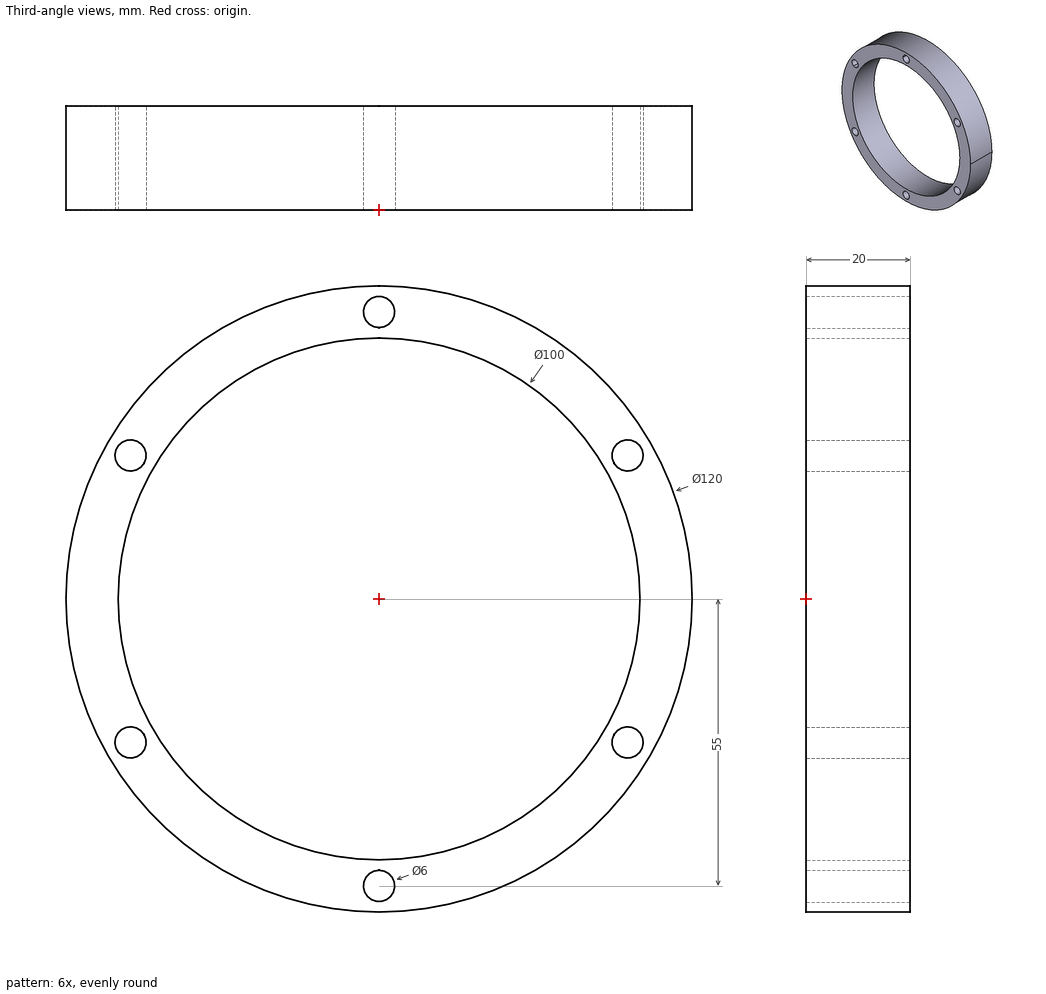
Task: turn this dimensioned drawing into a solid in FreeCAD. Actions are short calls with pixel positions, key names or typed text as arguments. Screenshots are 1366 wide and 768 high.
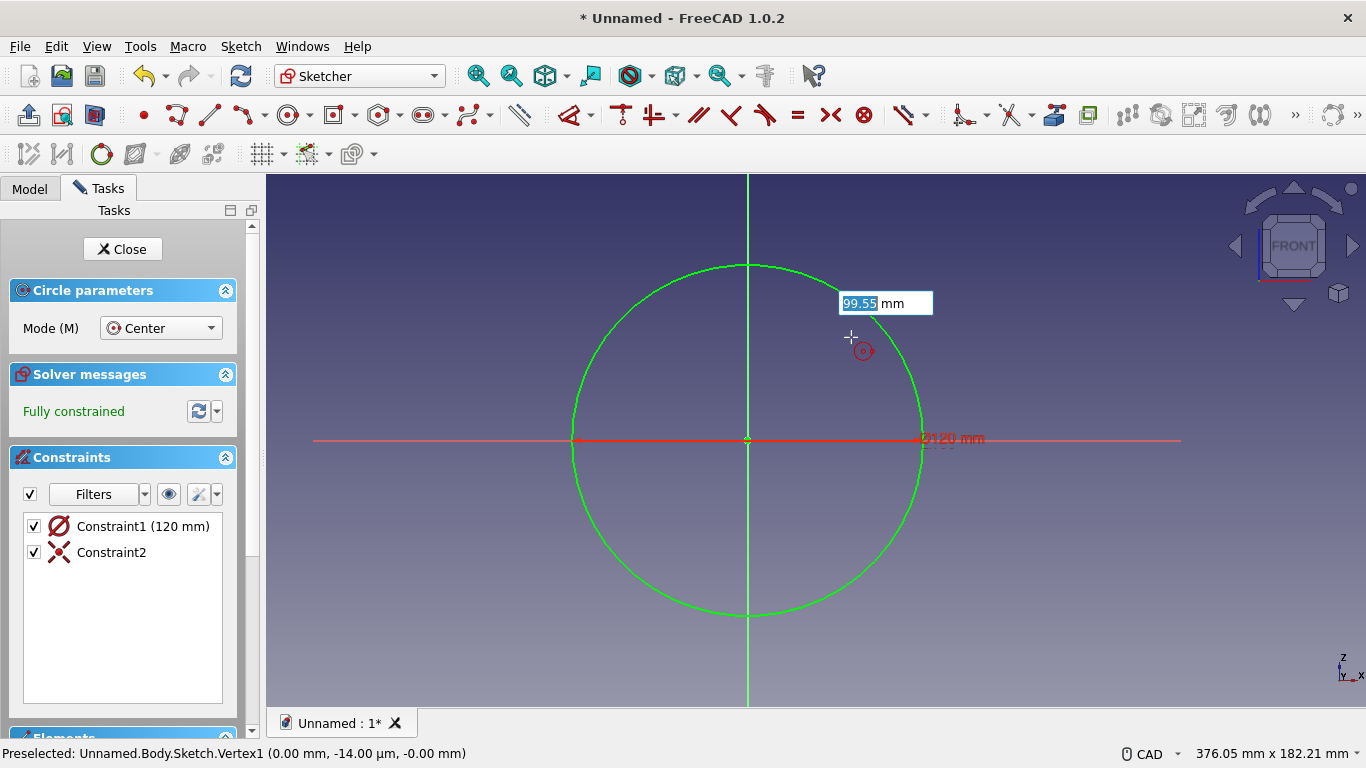
text(100)
key(Return)
key(Escape)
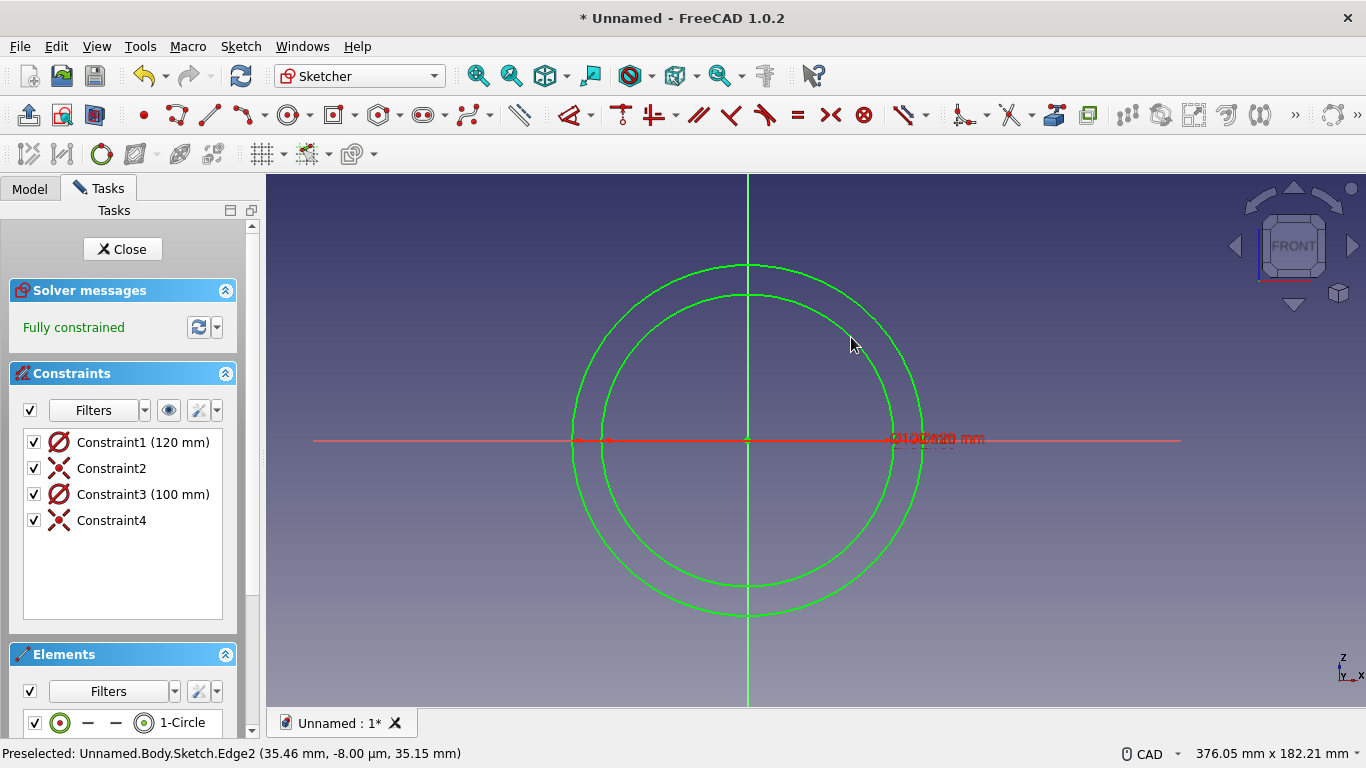
click(123, 249)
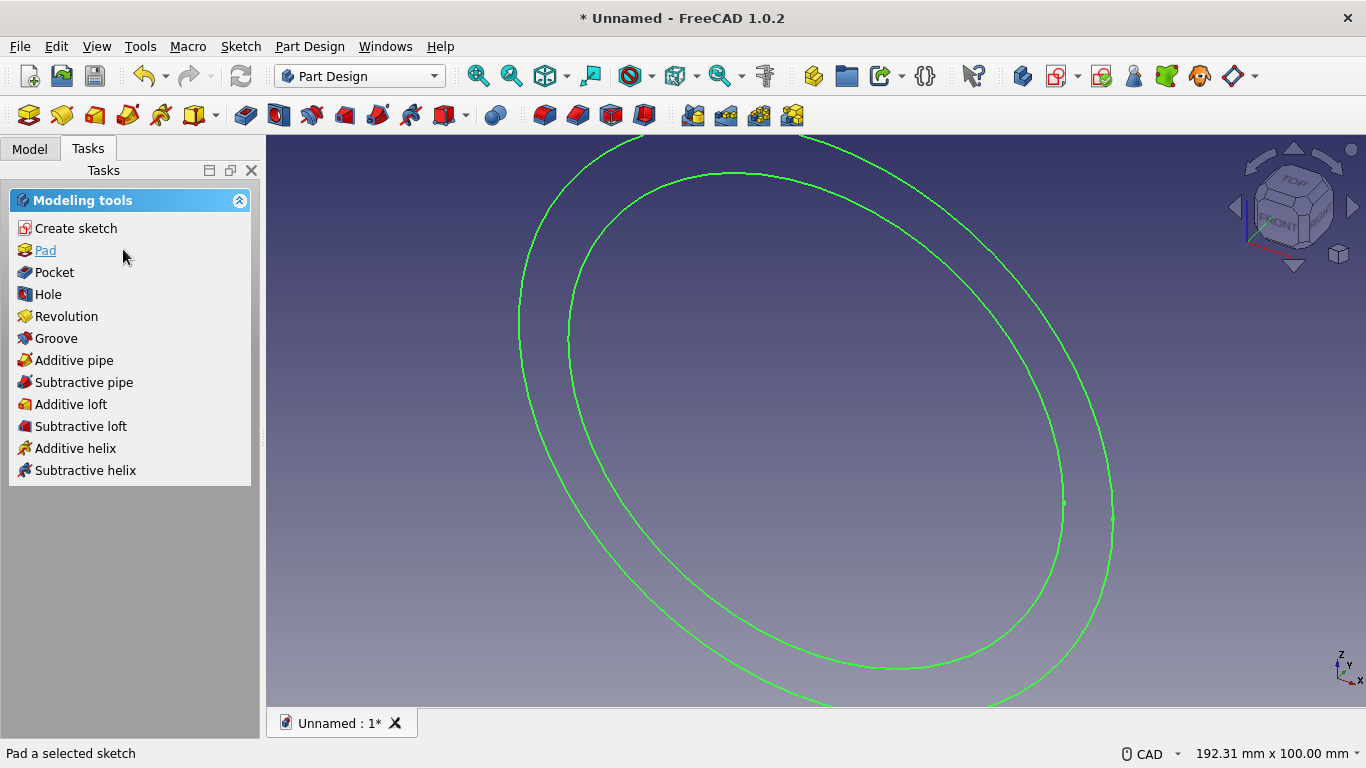
click(29, 116)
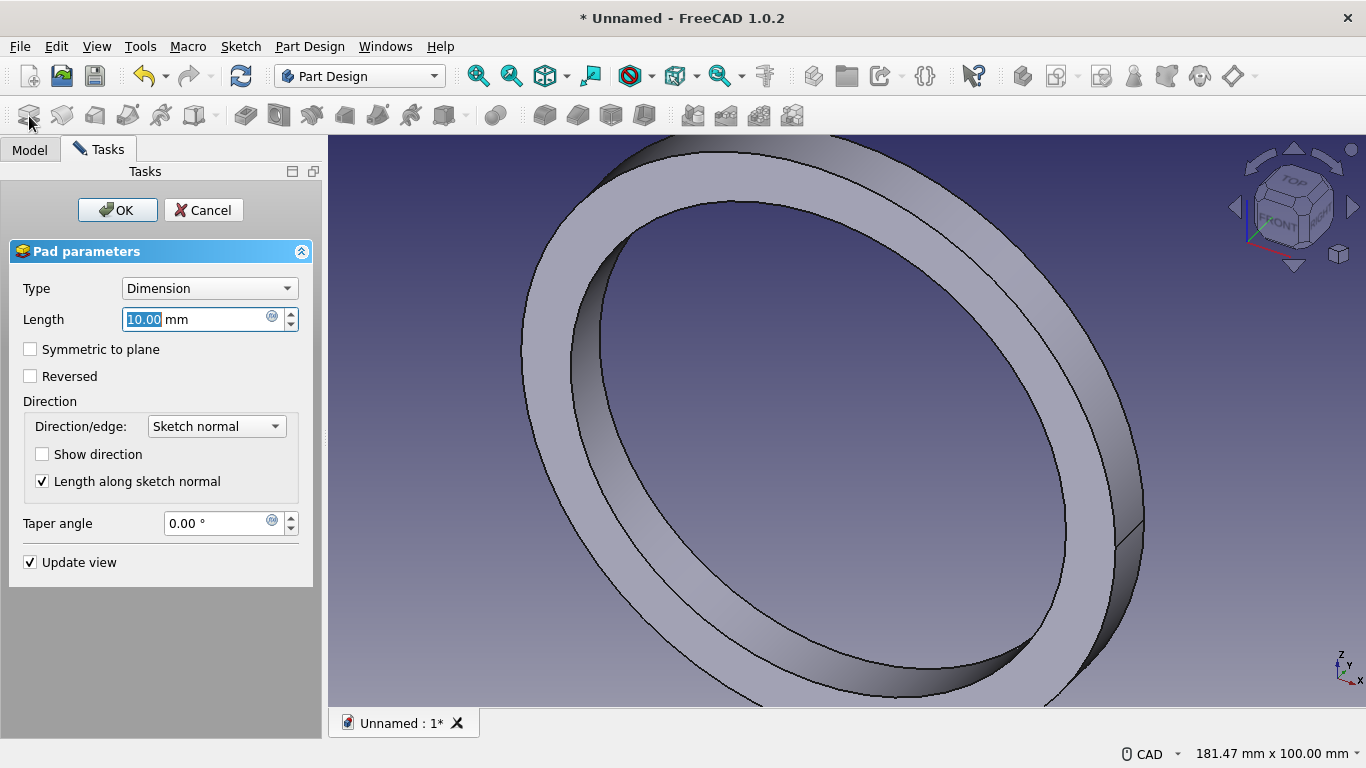
text(20)
key(Tab)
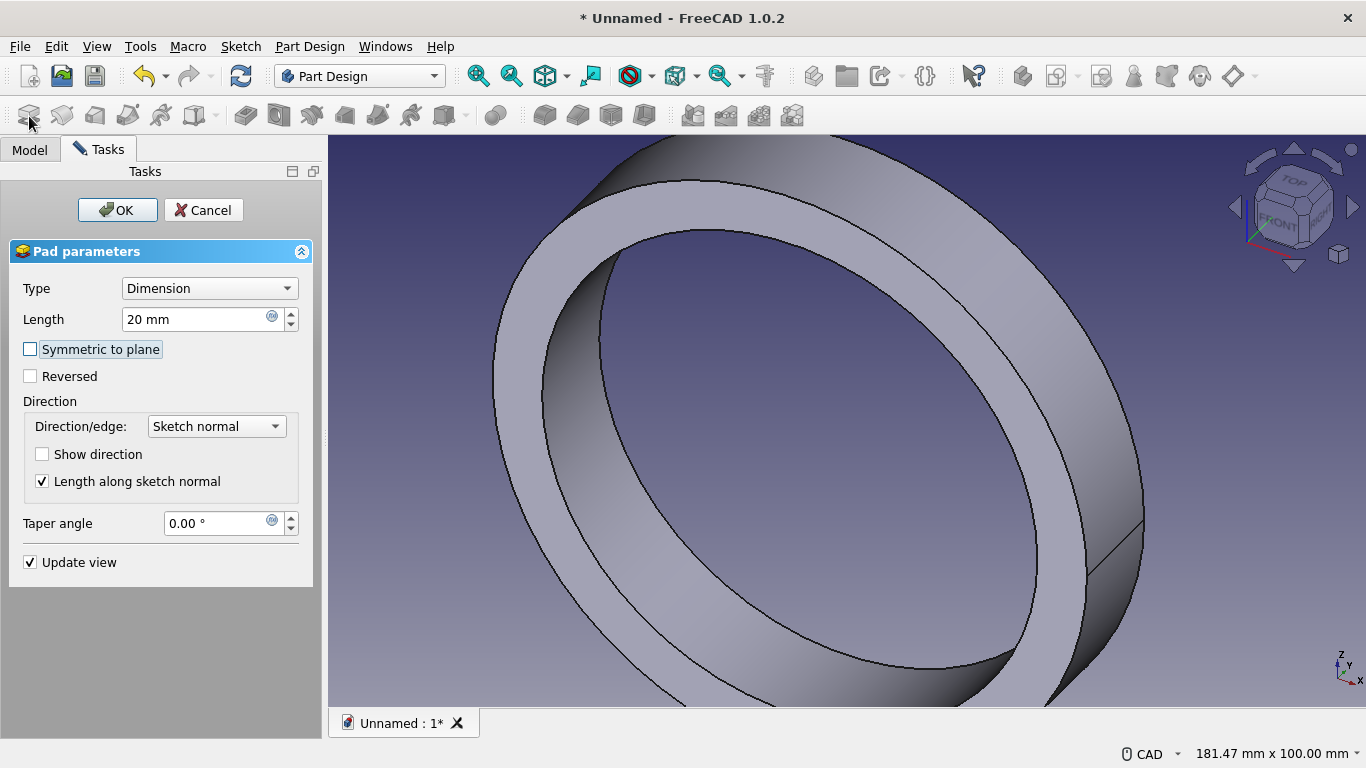
click(31, 376)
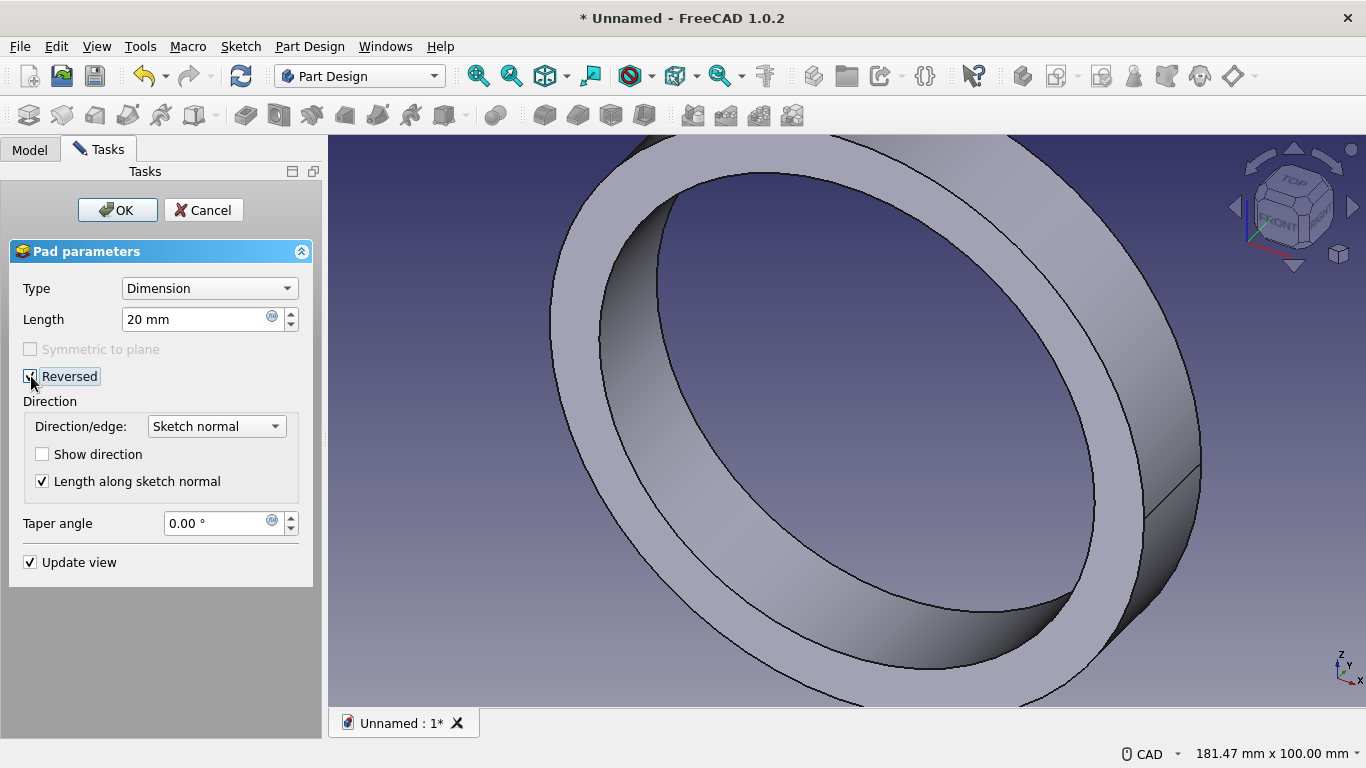
click(118, 210)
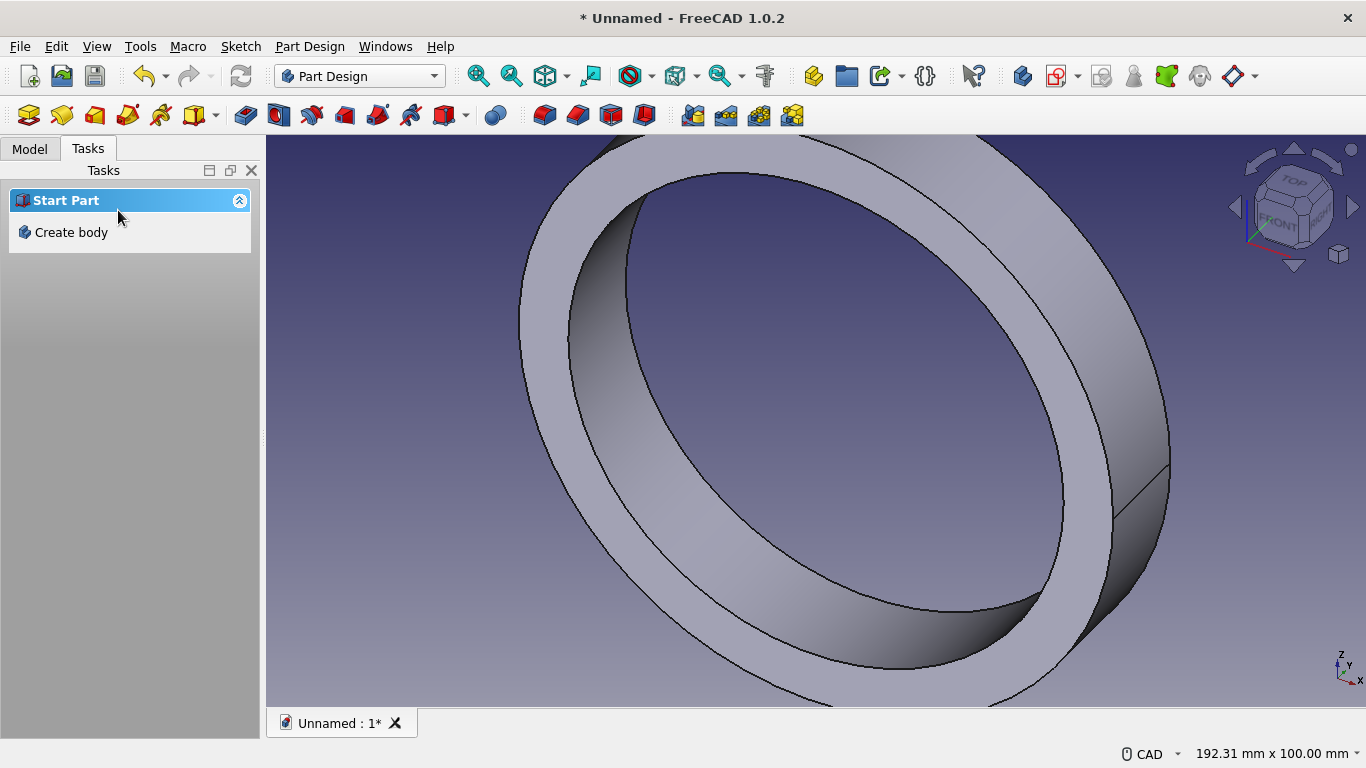
click(479, 76)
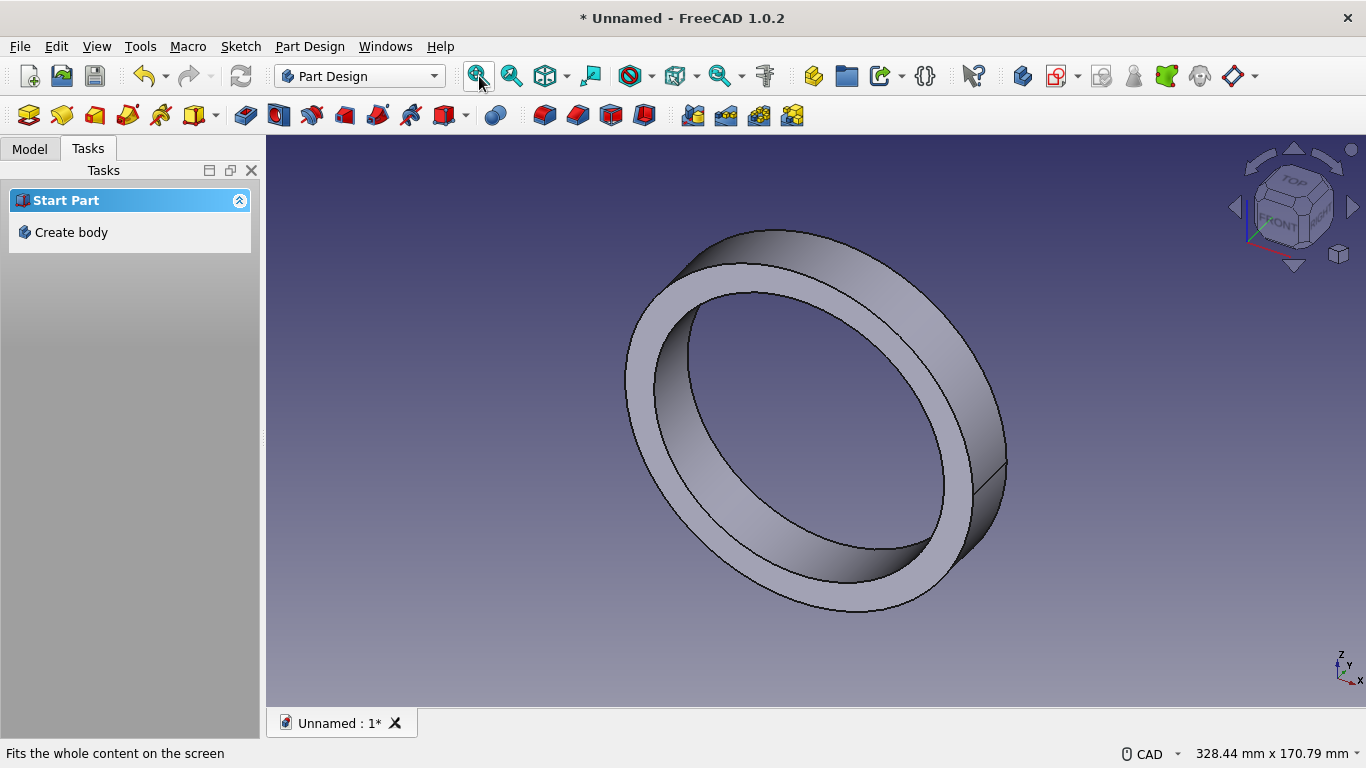
key(4)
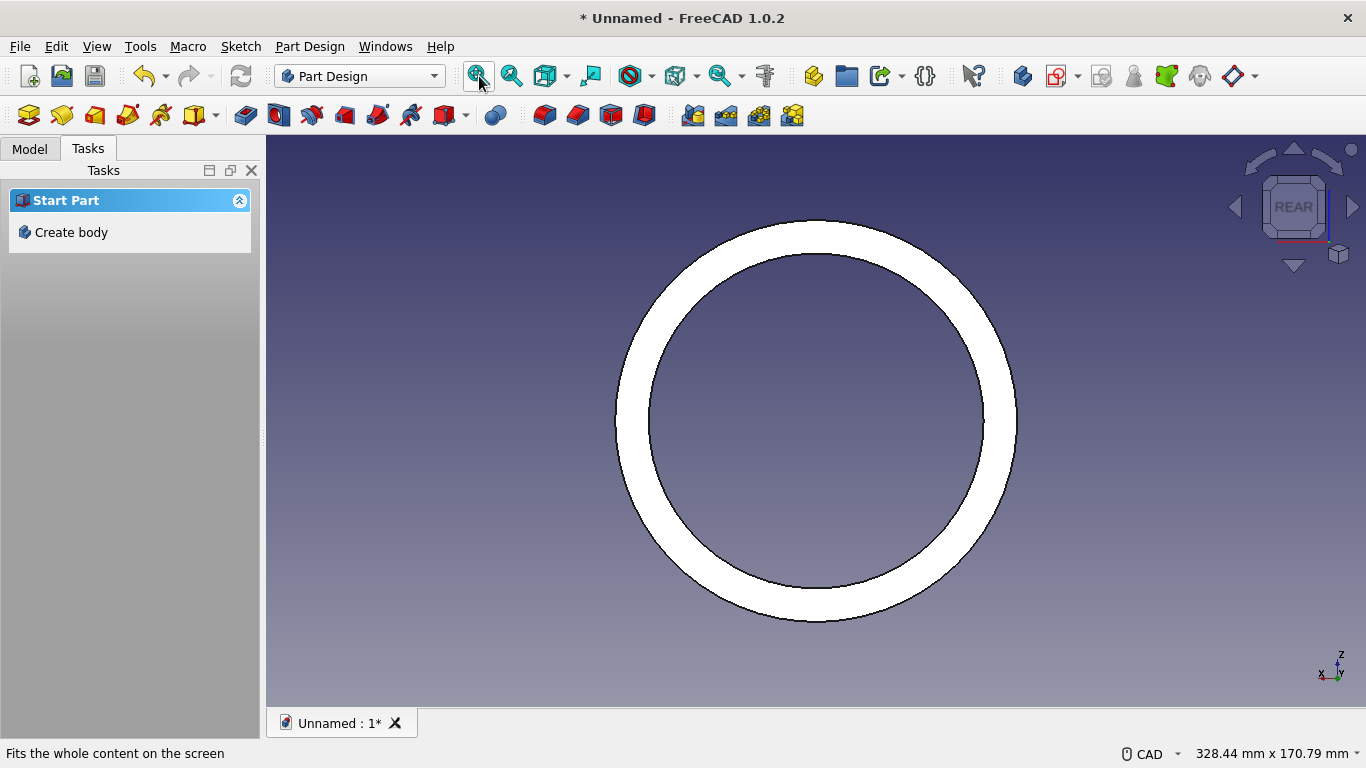
click(874, 248)